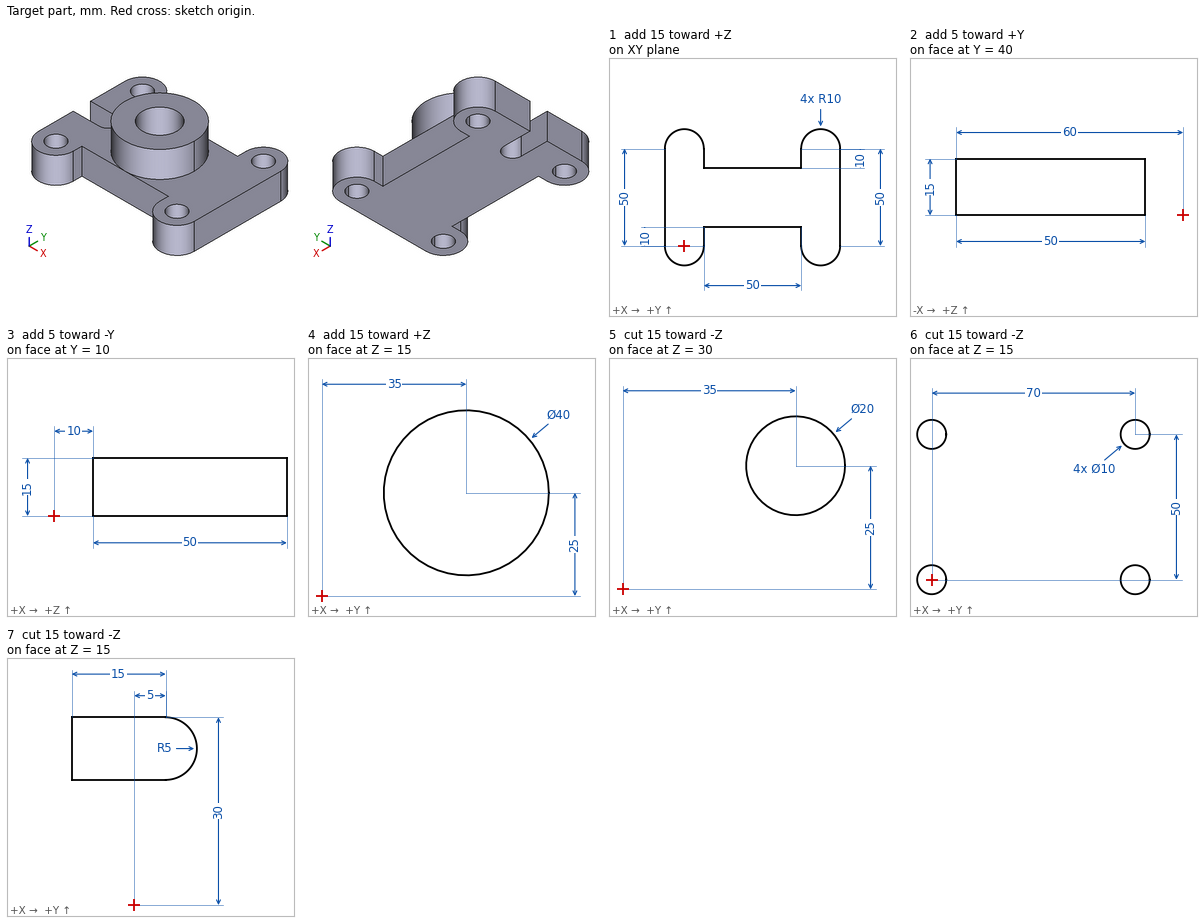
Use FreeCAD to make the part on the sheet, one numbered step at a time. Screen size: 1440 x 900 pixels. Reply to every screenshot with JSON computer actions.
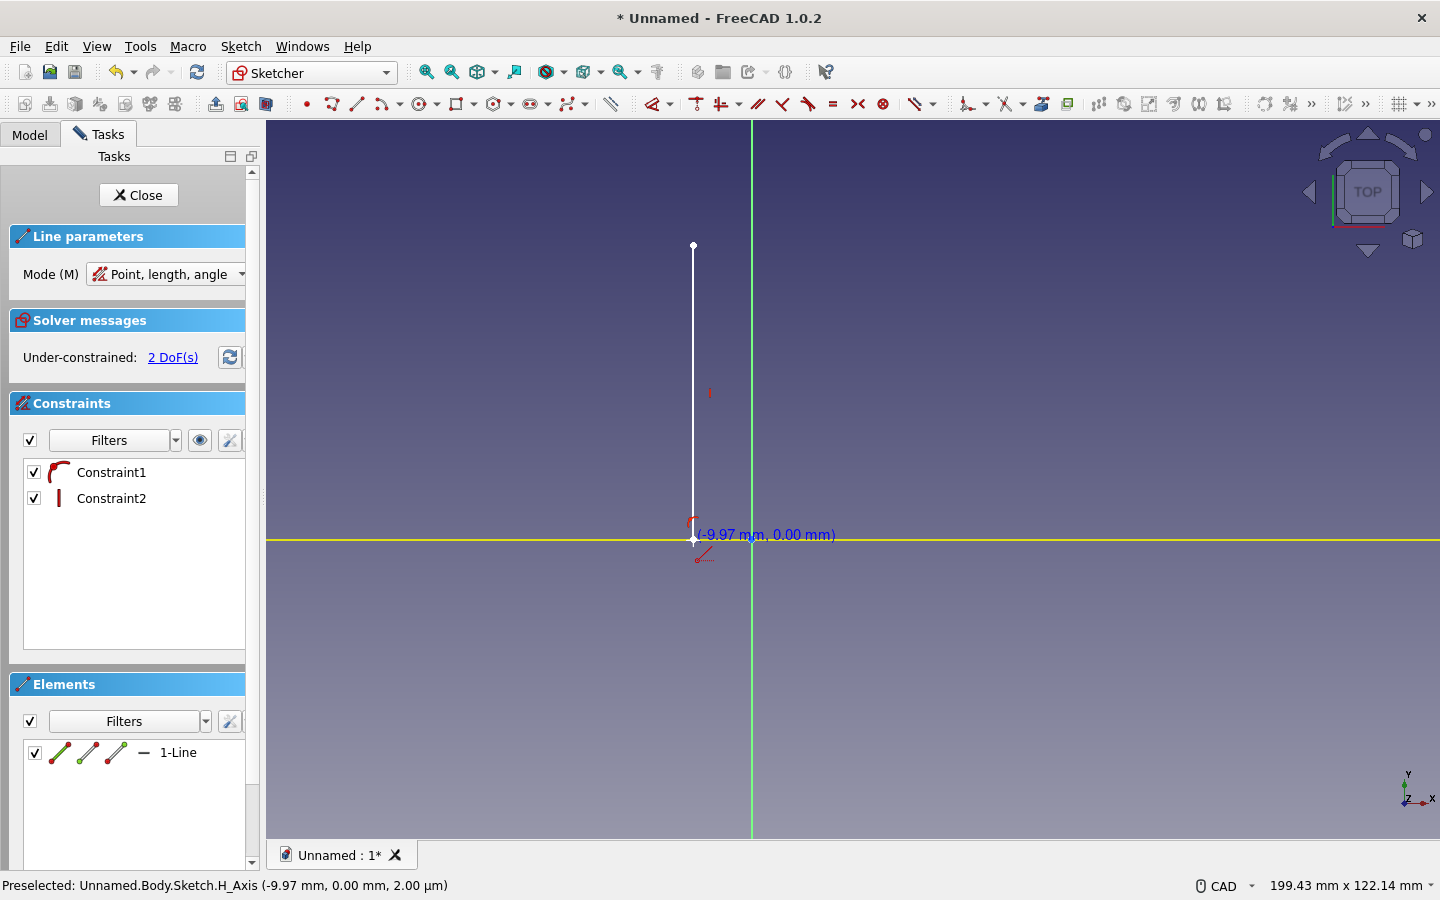
{"action": "left_click", "coordinate": [332, 104]}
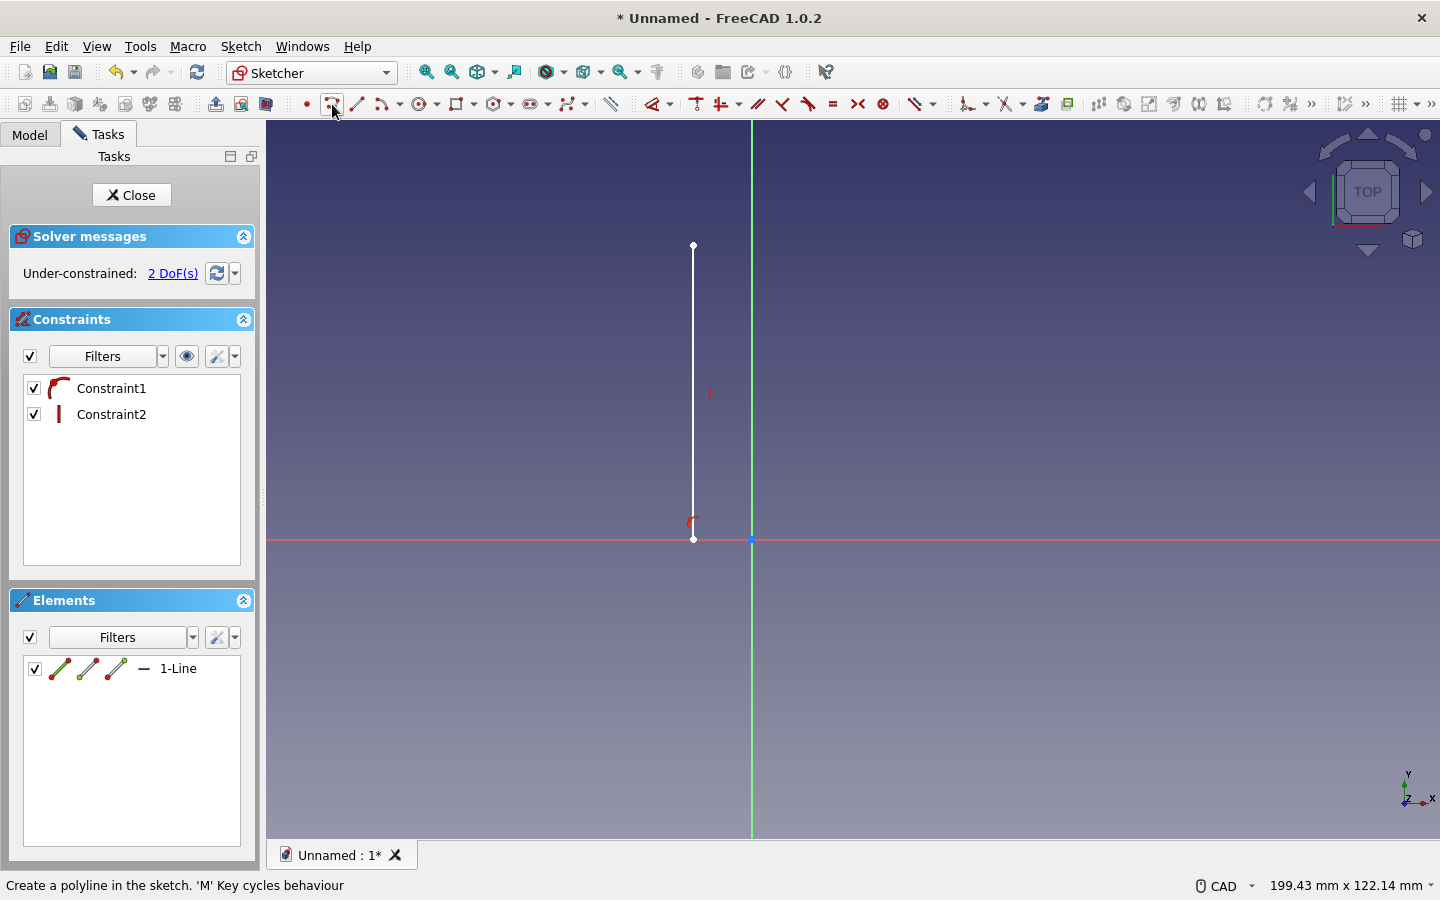
{"action": "left_click", "coordinate": [811, 540]}
{"action": "left_click", "coordinate": [811, 481]}
{"action": "left_click", "coordinate": [1105, 481]}
{"action": "left_click", "coordinate": [1105, 540]}
{"action": "right_click", "coordinate": [1105, 540]}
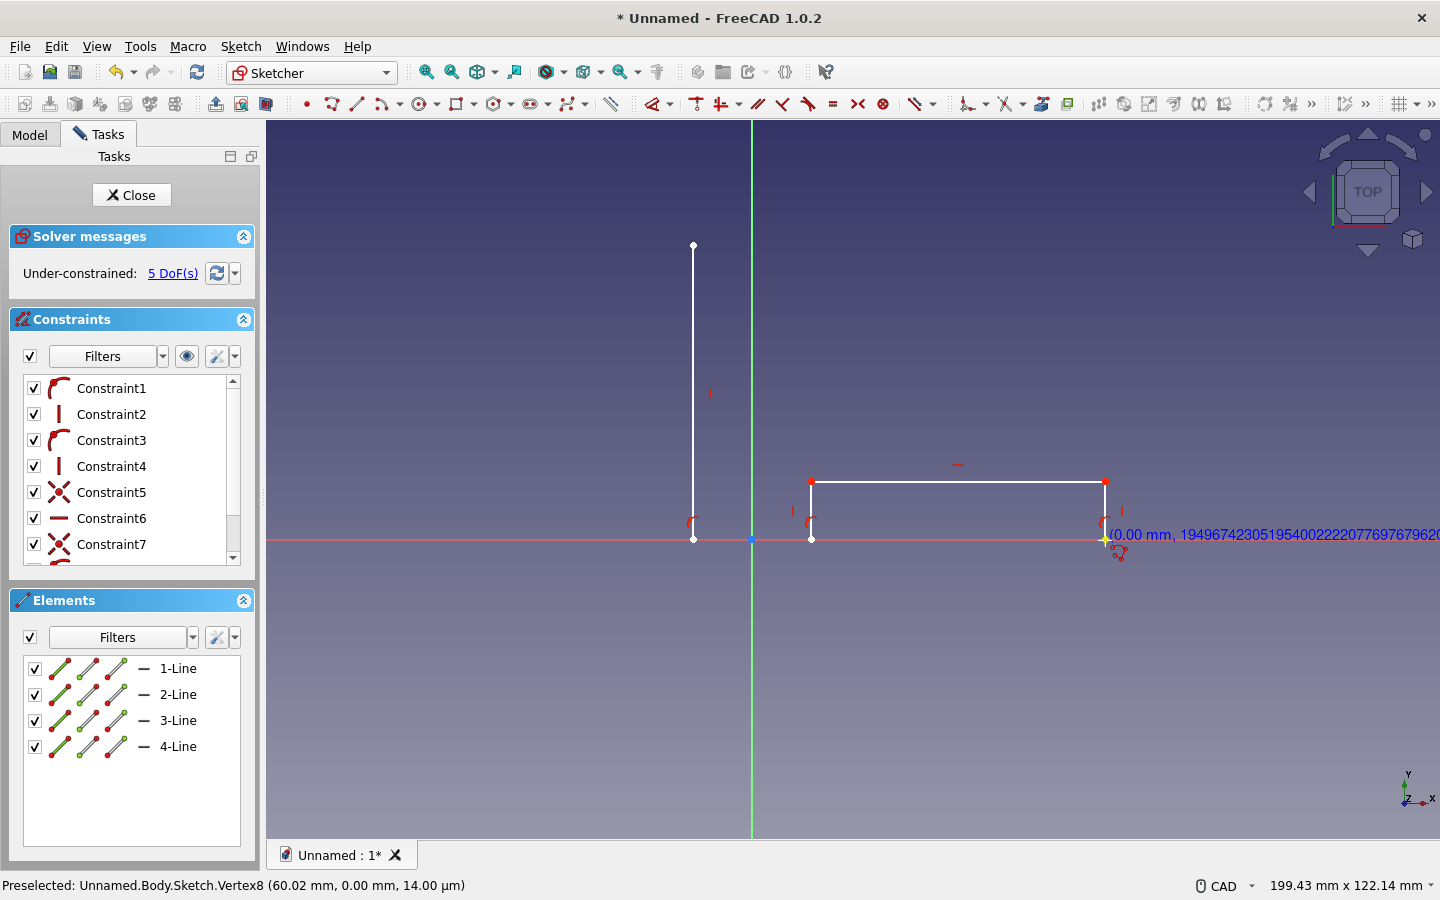
{"action": "left_click", "coordinate": [357, 104]}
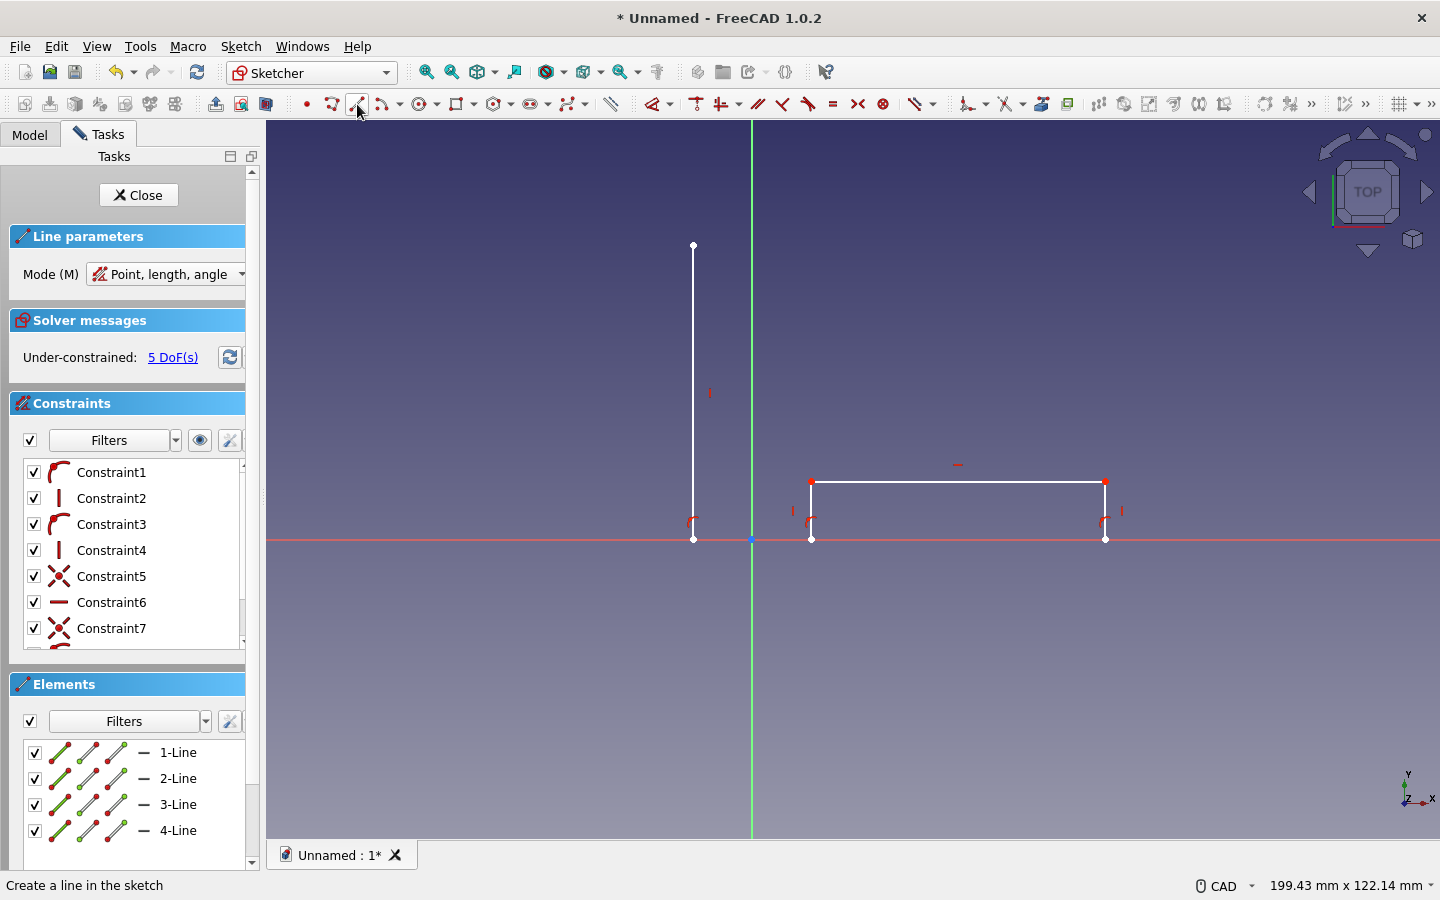
{"action": "left_click", "coordinate": [1223, 540]}
{"action": "left_click", "coordinate": [1223, 245]}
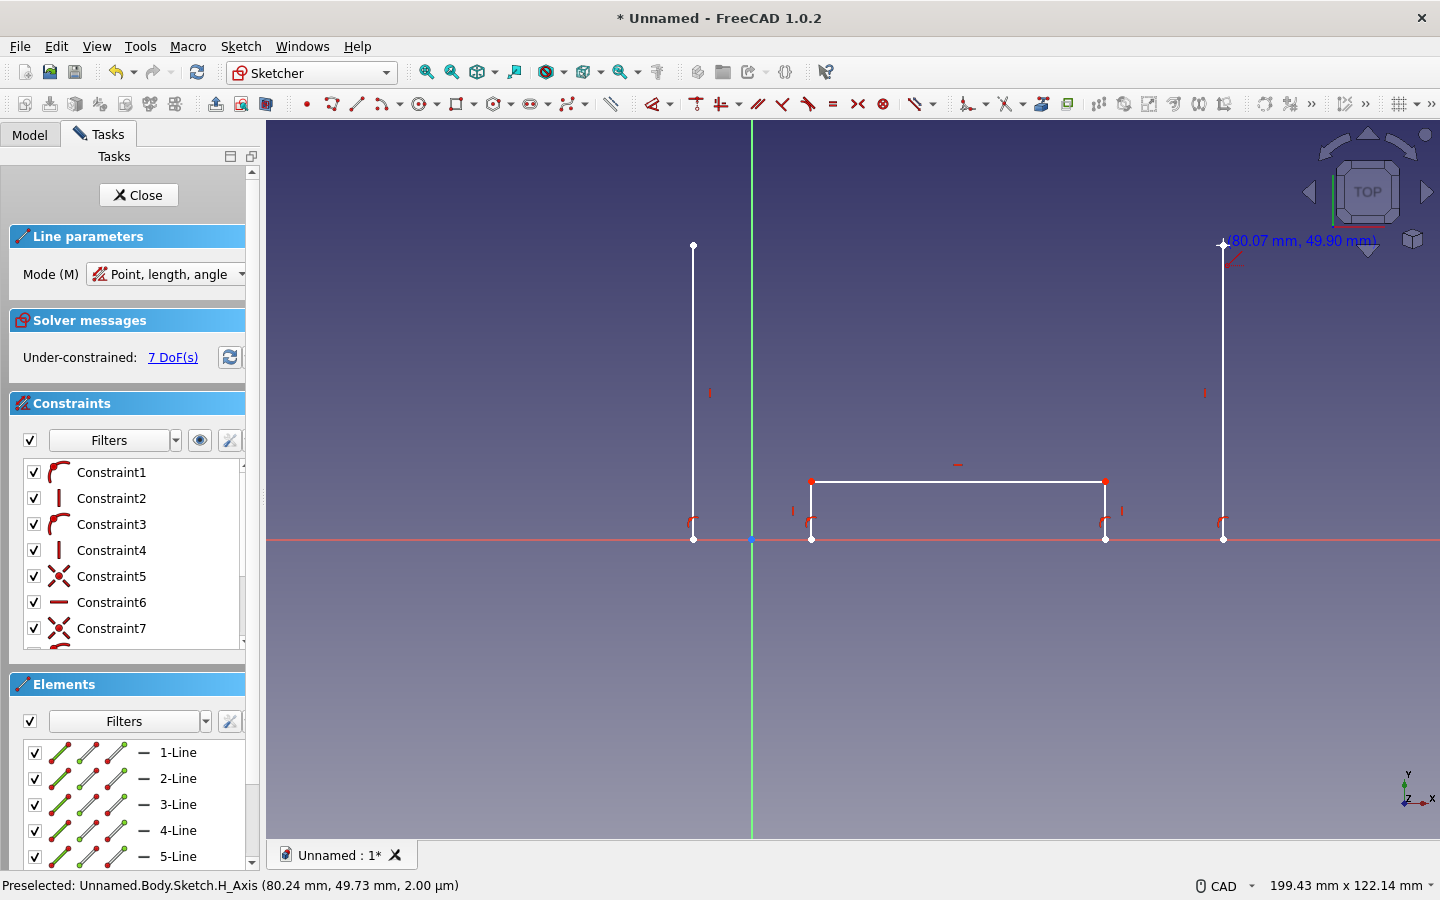
{"action": "key", "text": "g m"}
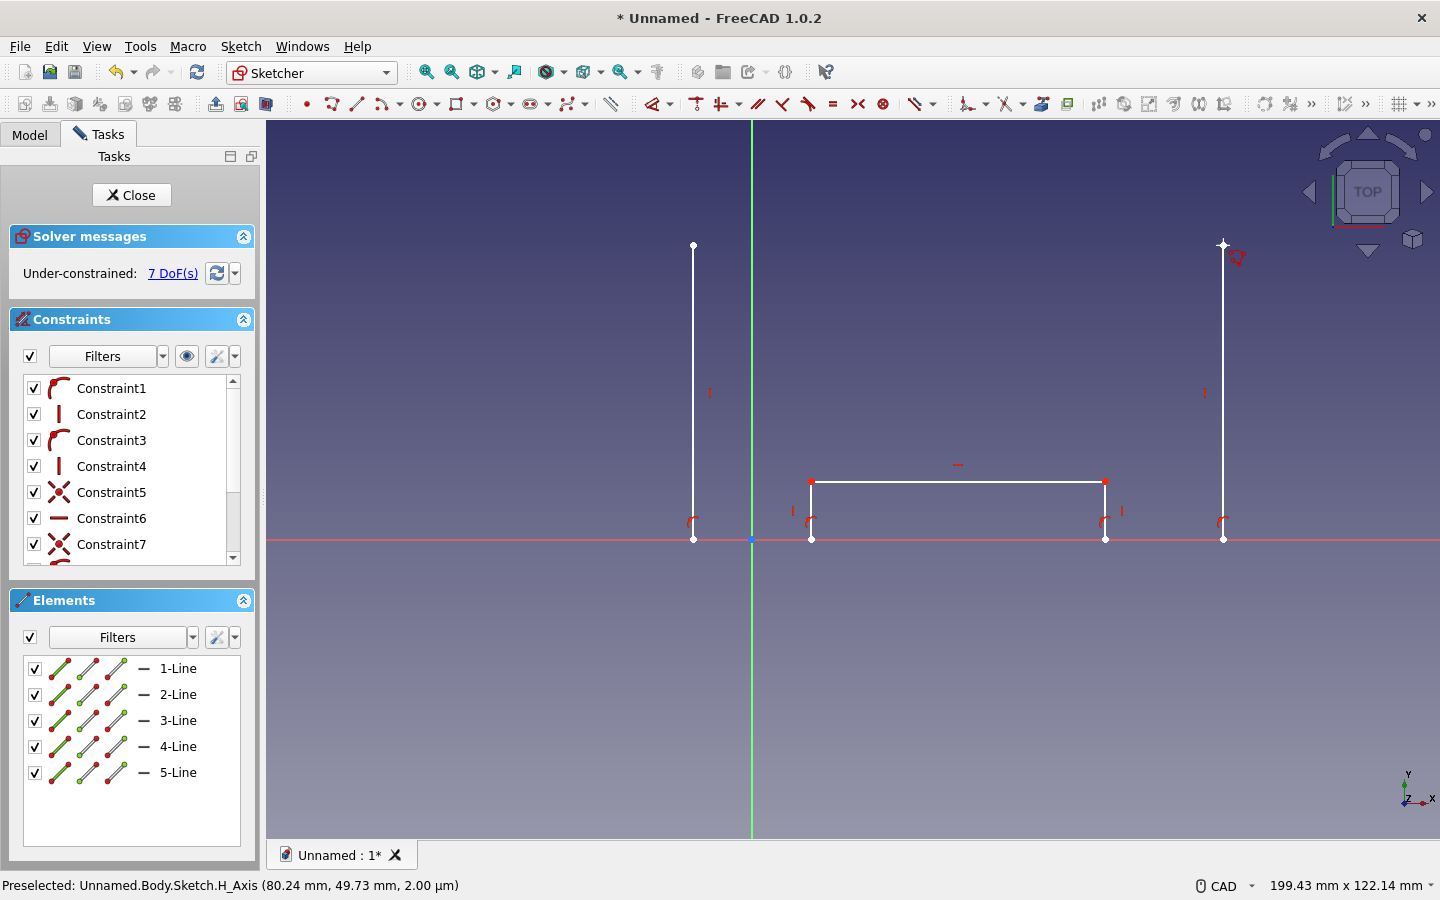
{"action": "left_click", "coordinate": [1105, 245]}
{"action": "left_click", "coordinate": [1105, 304]}
{"action": "left_click", "coordinate": [811, 304]}
{"action": "left_click", "coordinate": [811, 245]}
{"action": "right_click", "coordinate": [811, 245]}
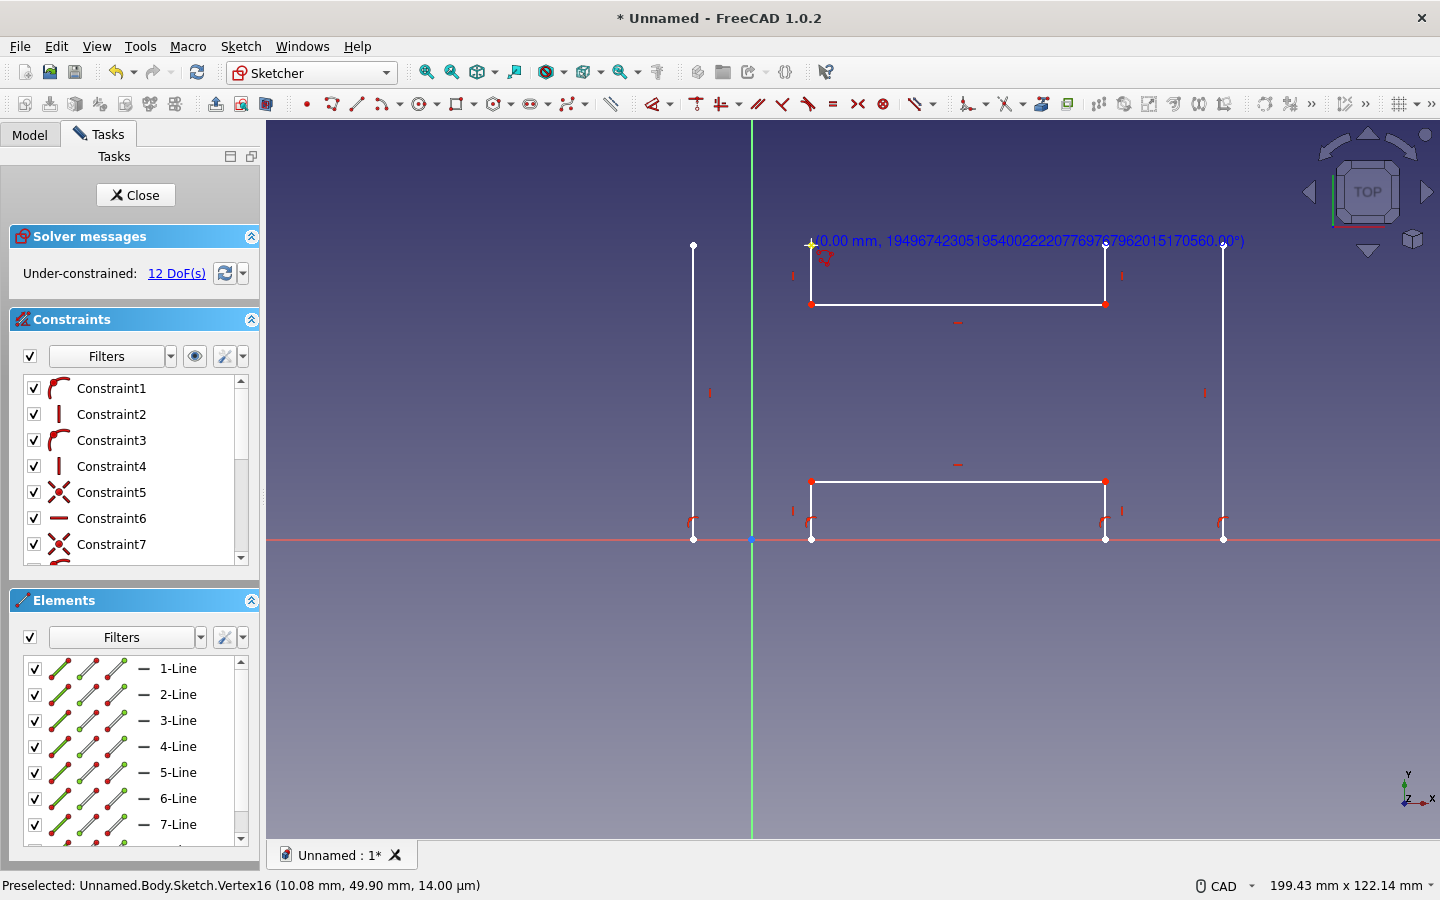
{"action": "left_click", "coordinate": [400, 104]}